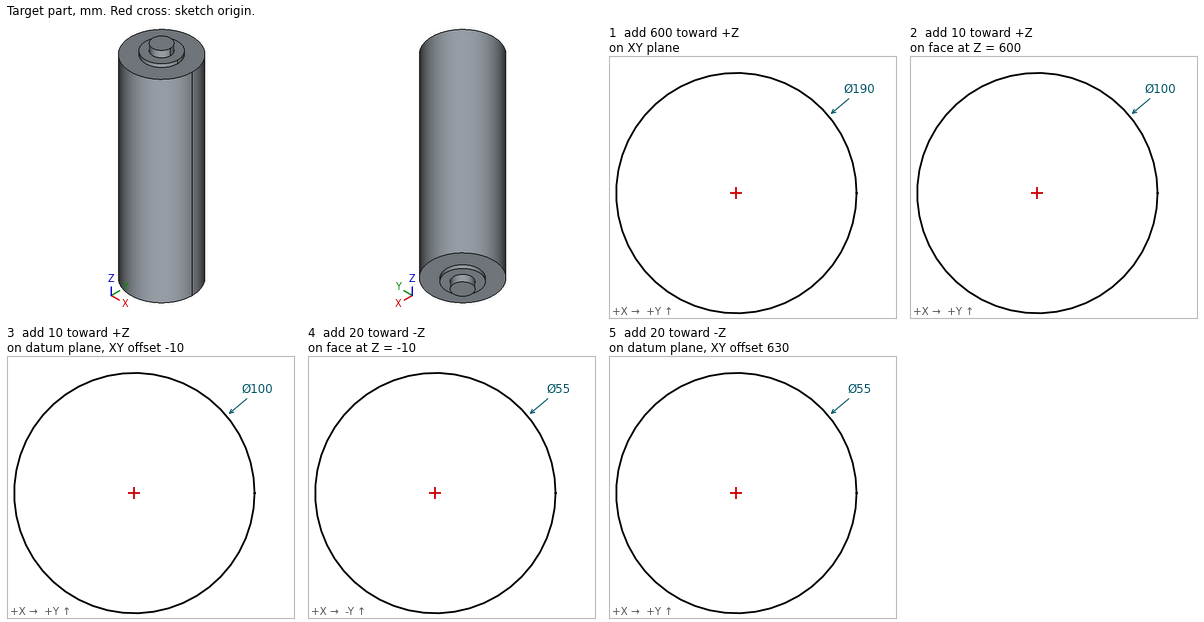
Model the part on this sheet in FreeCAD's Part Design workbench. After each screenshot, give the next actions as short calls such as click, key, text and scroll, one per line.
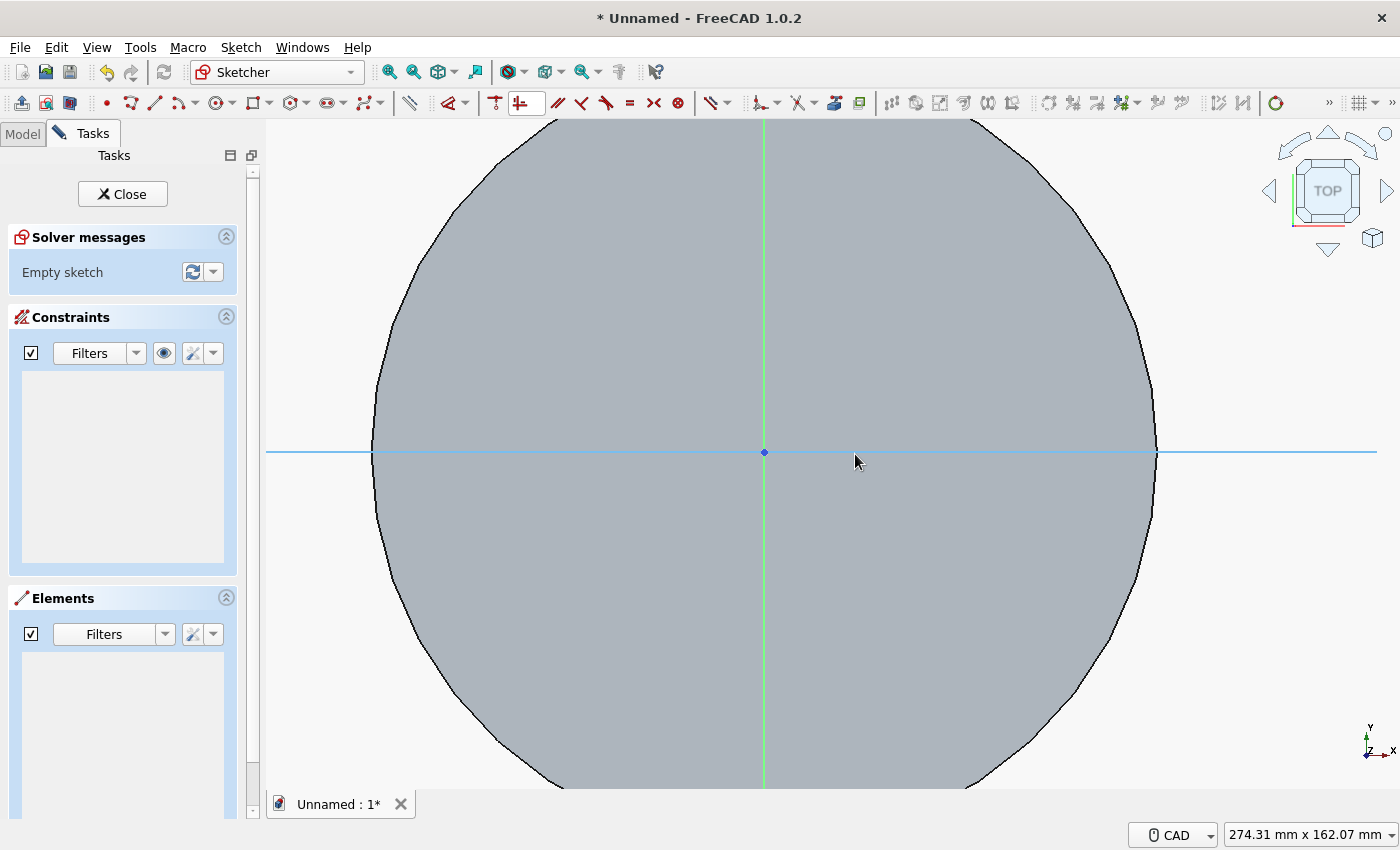
click(216, 104)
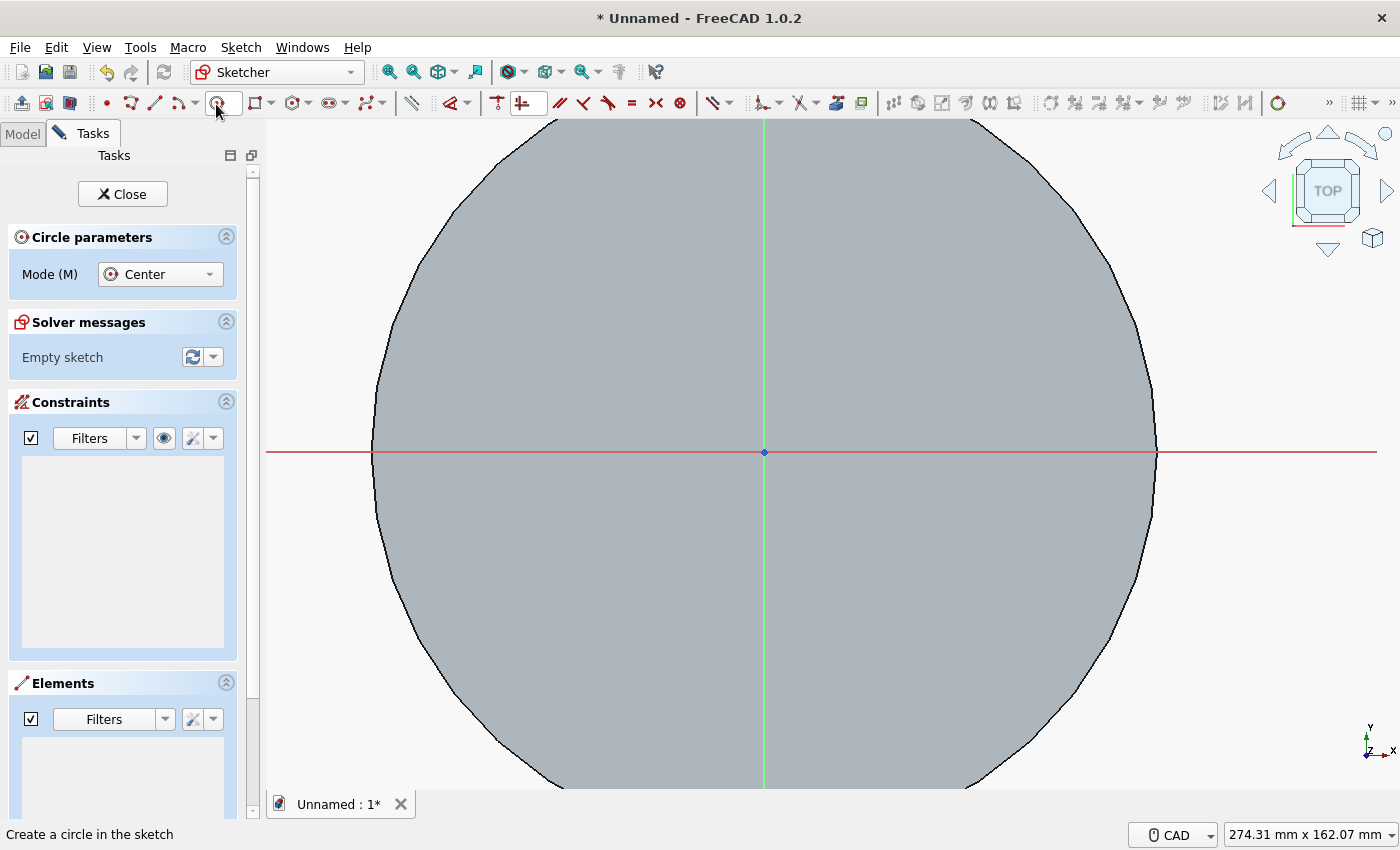
click(764, 452)
click(910, 306)
key(Escape)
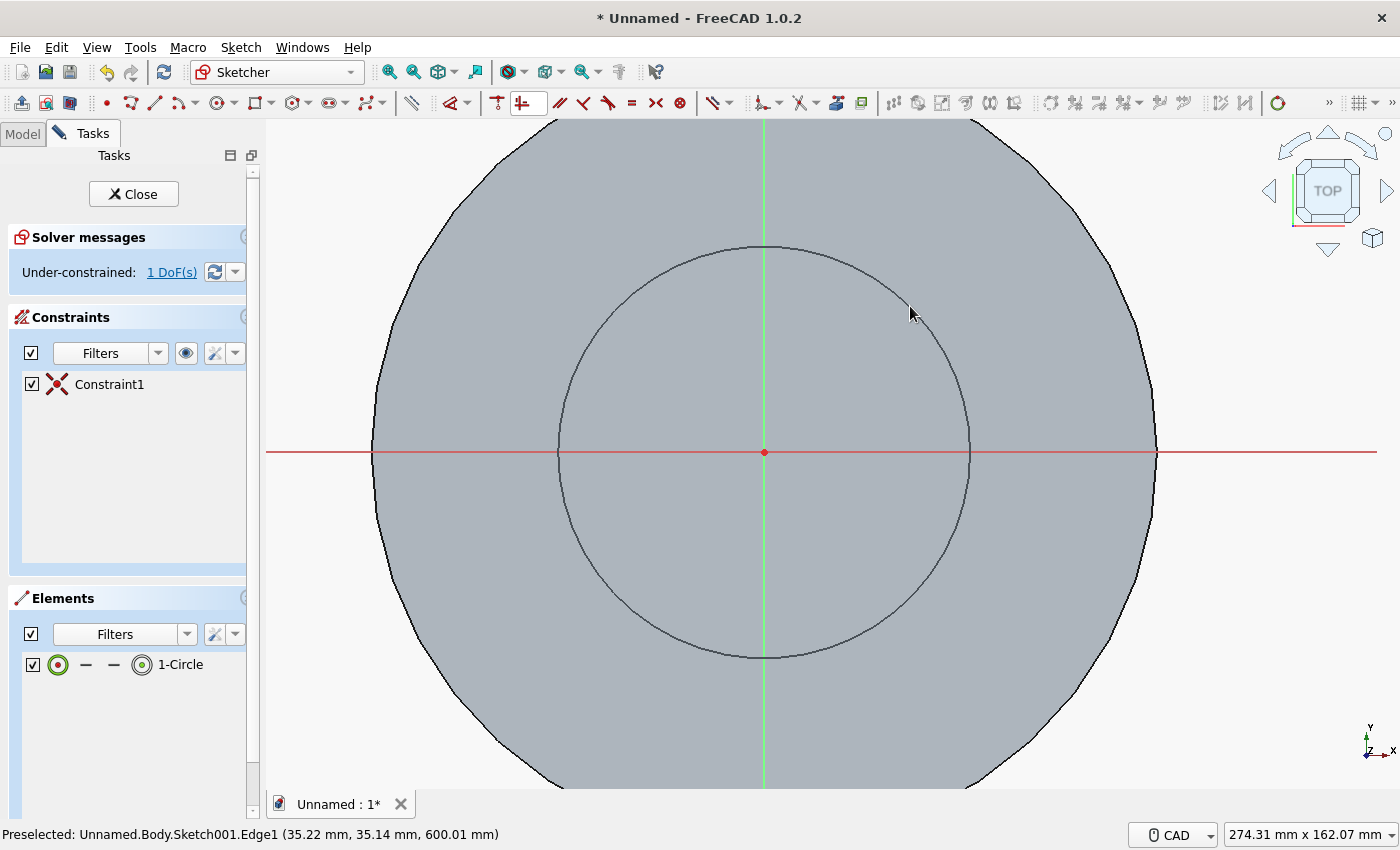
click(450, 104)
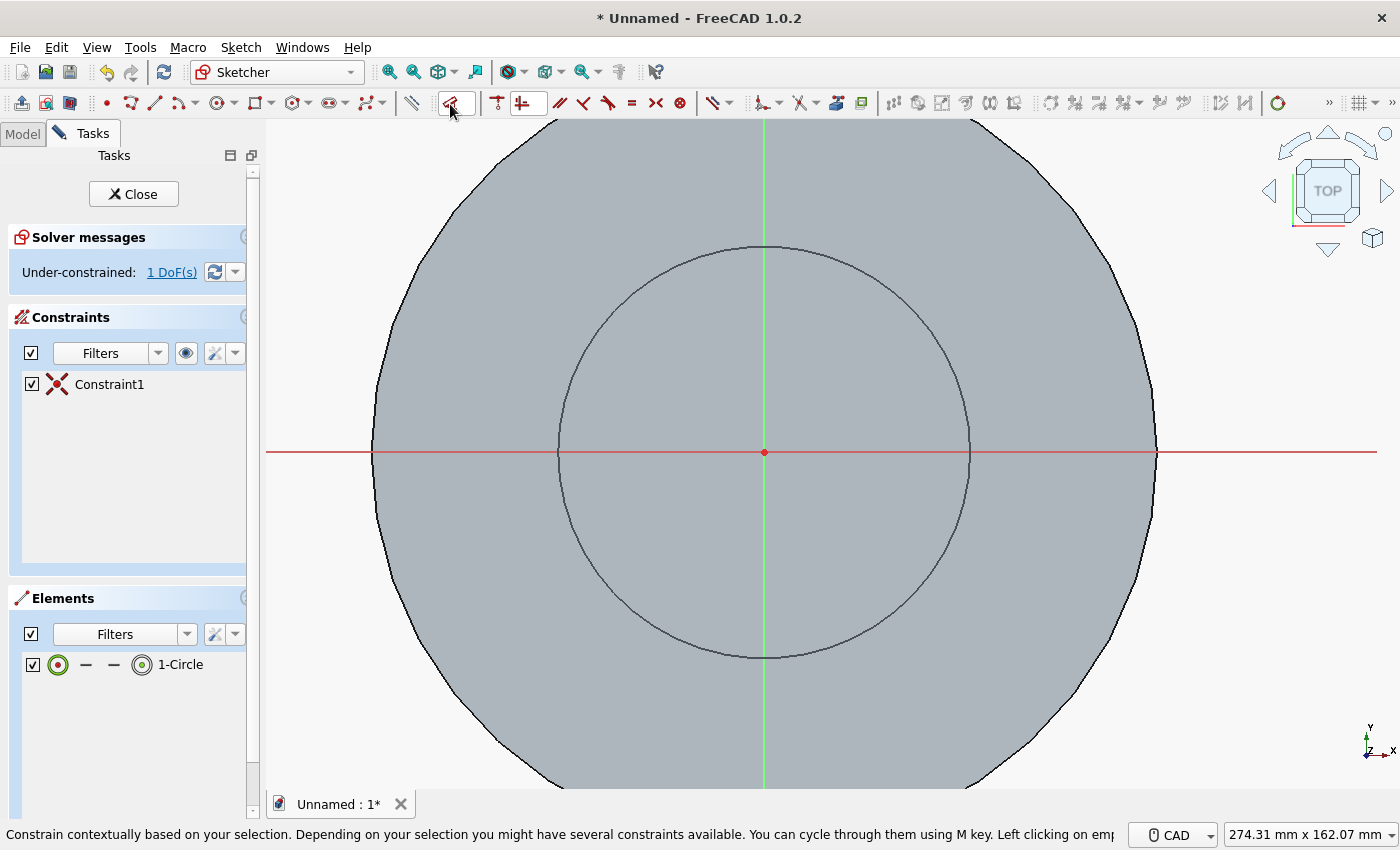
click(909, 306)
click(931, 283)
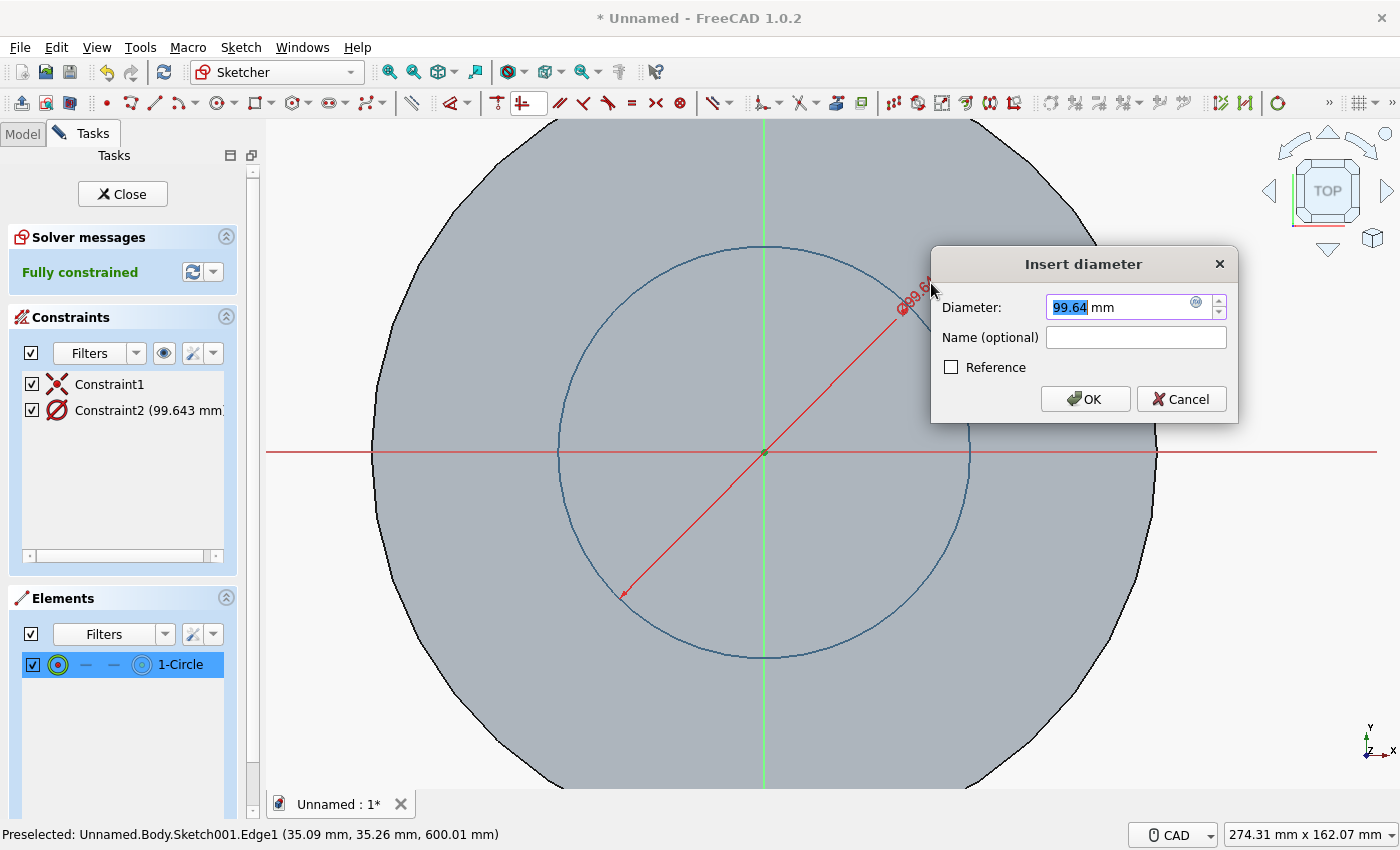
text(100)
key(Return)
key(Escape)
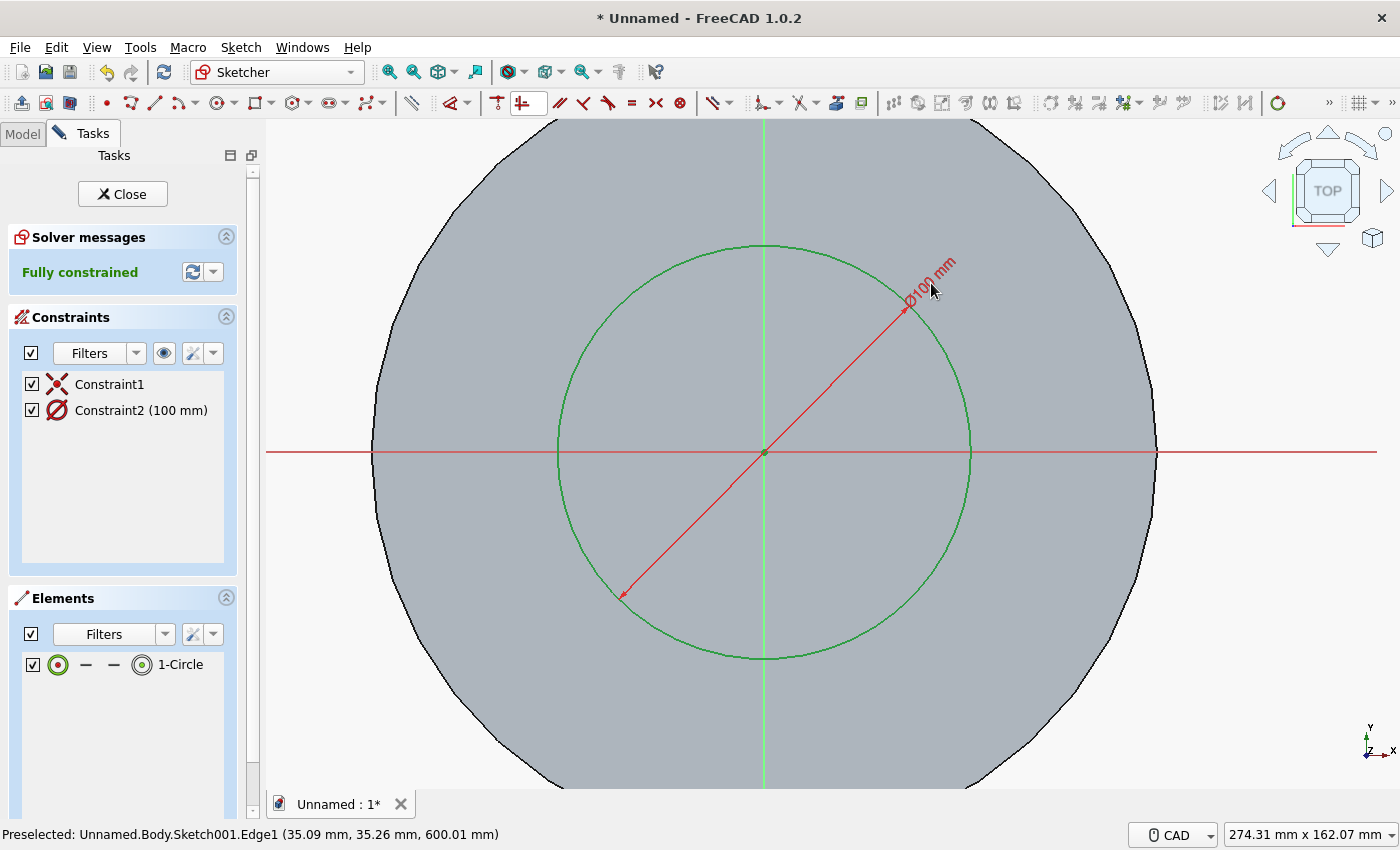
click(123, 194)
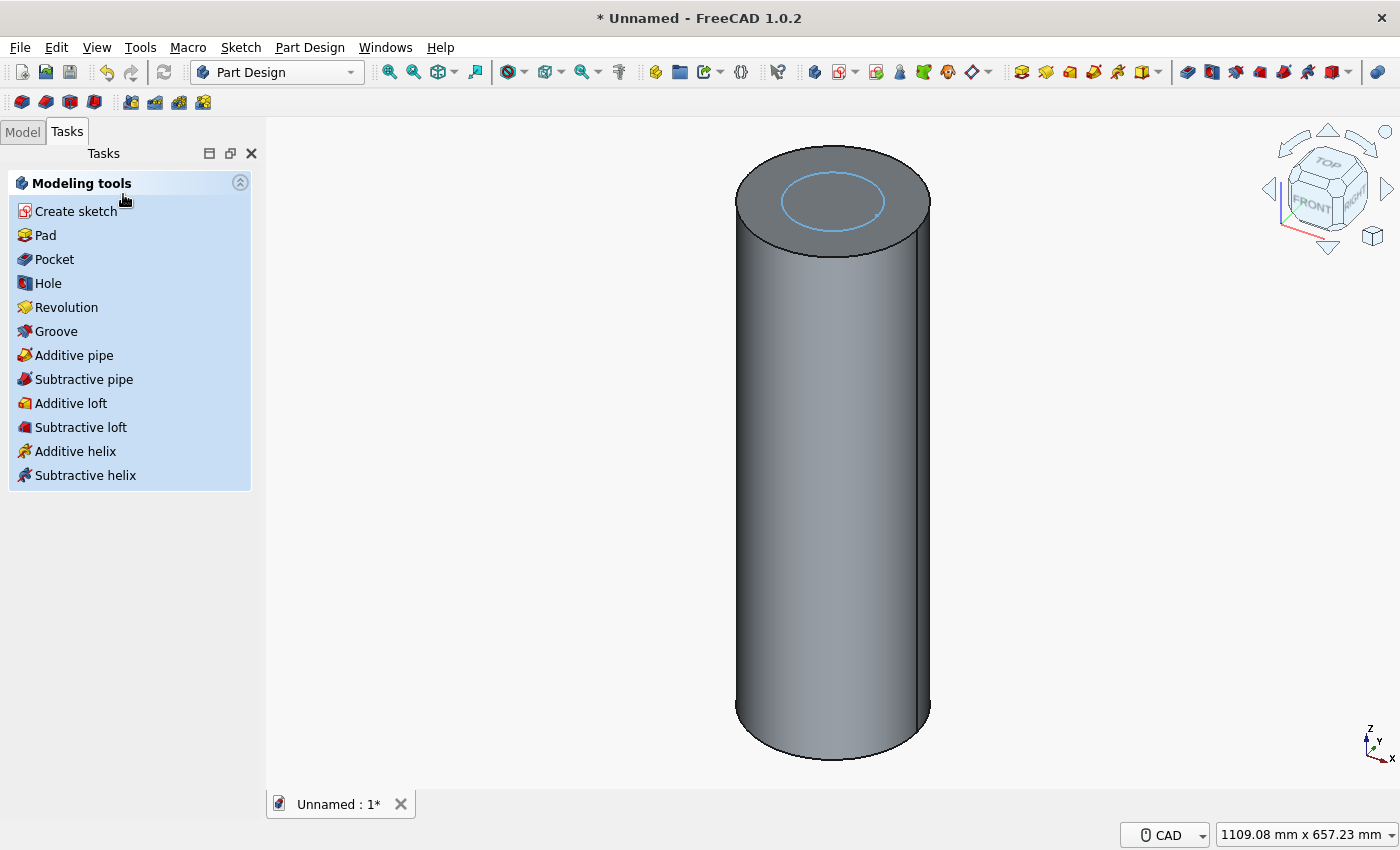
click(1022, 72)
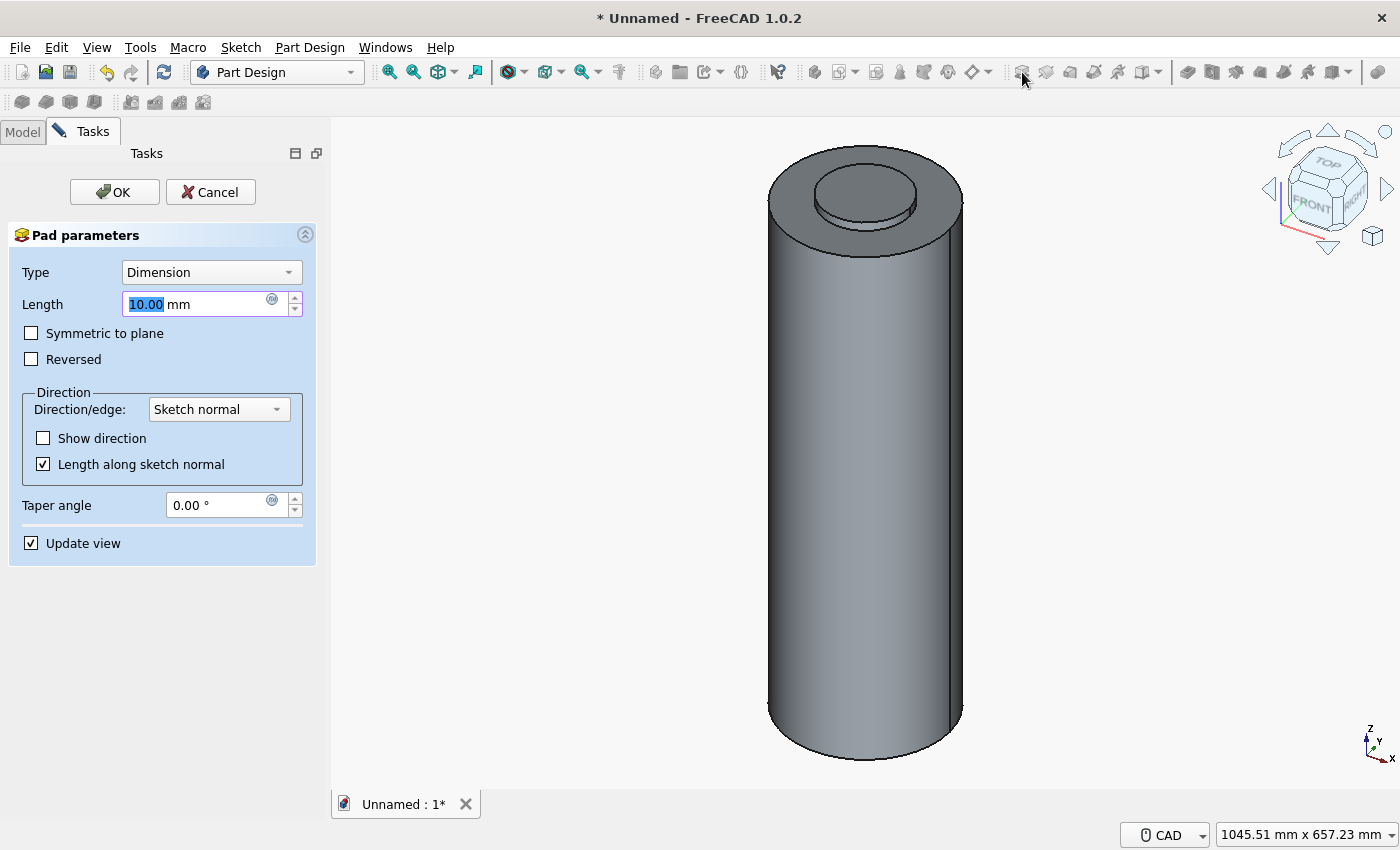
text(10)
key(Tab)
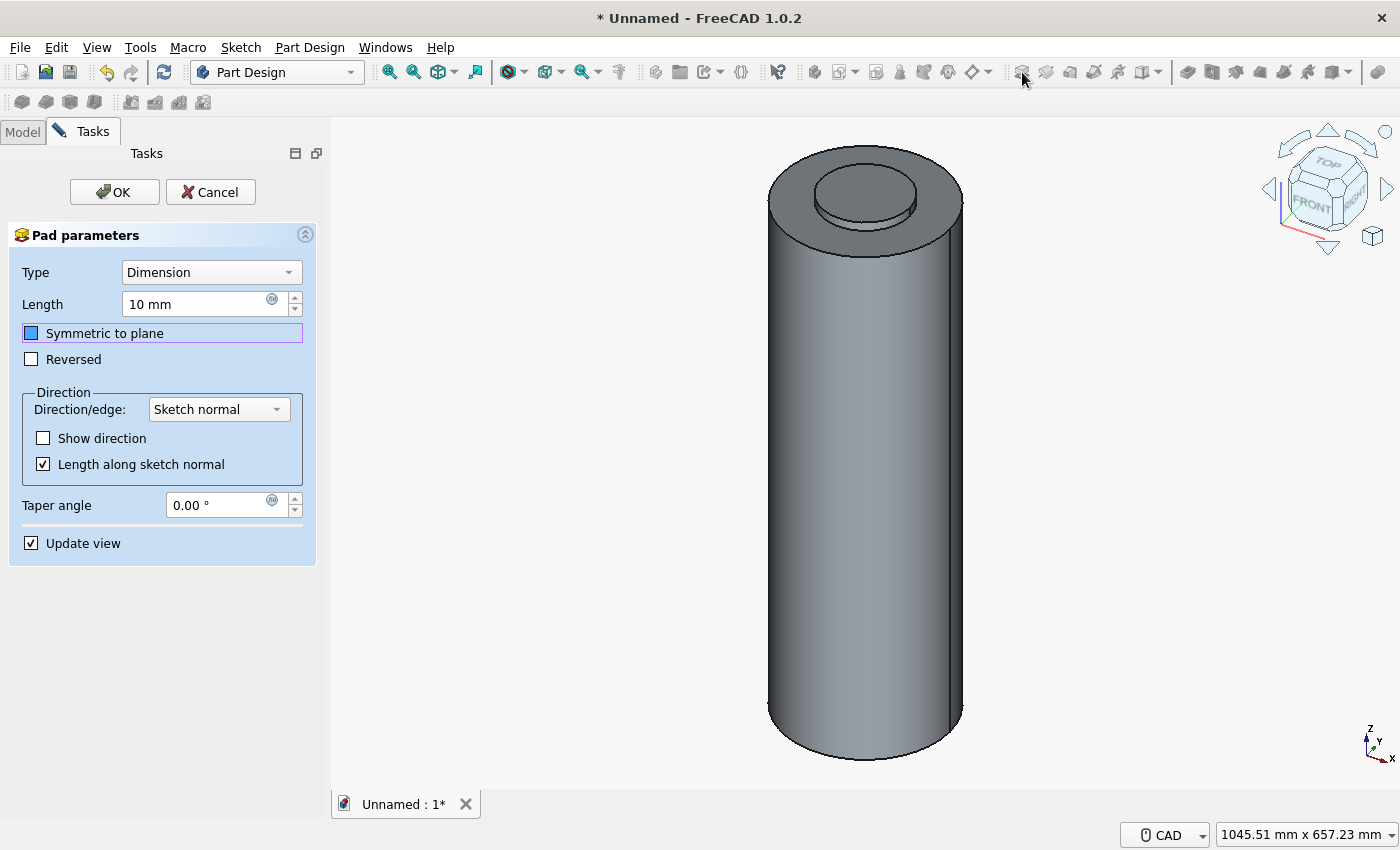
click(115, 192)